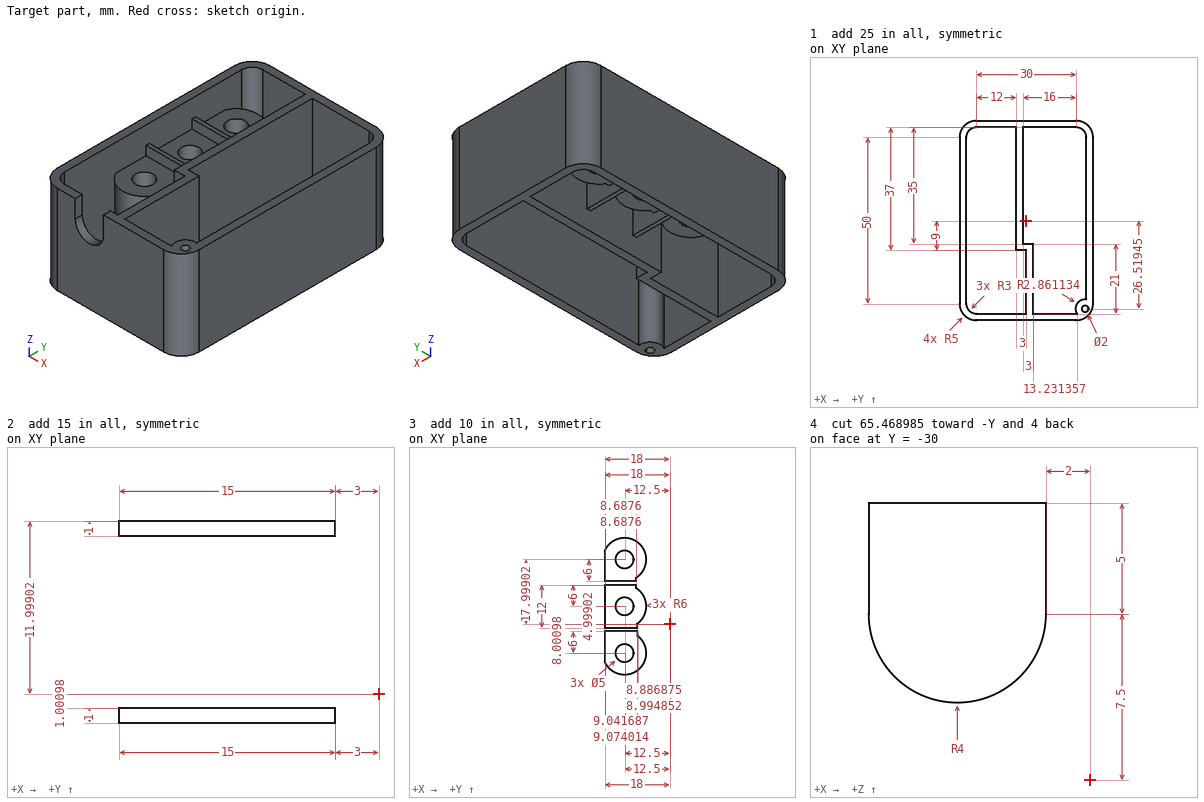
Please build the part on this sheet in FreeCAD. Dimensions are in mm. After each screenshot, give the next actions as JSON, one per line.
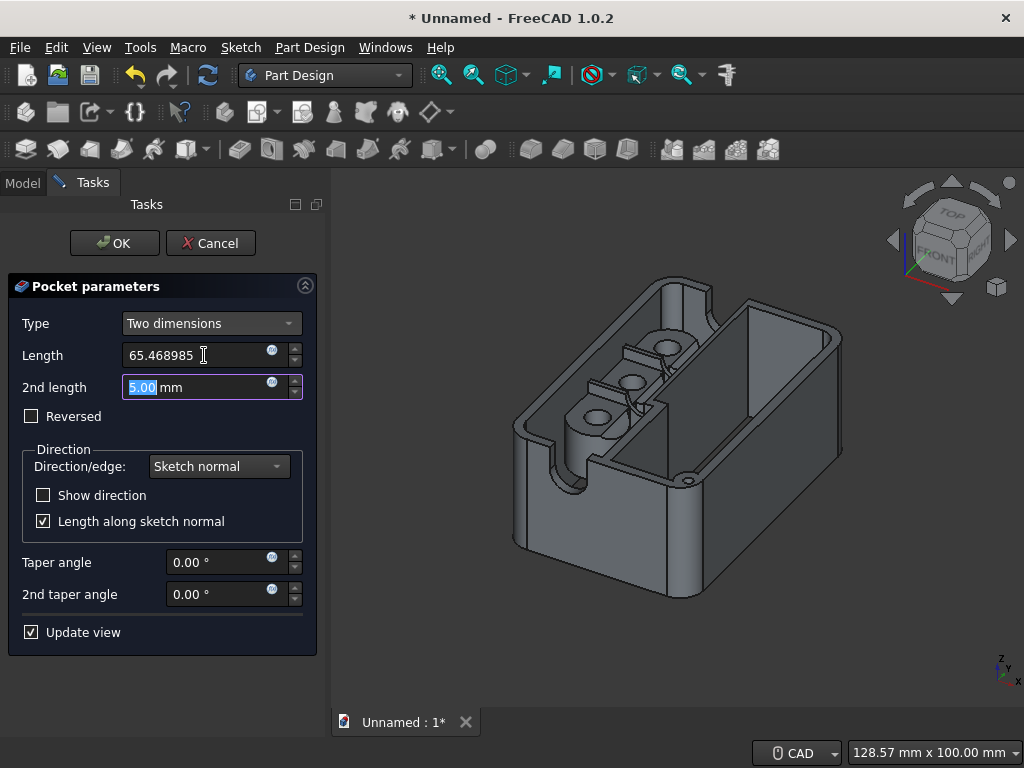
{"action": "type", "text": "4"}
{"action": "key", "text": "Tab"}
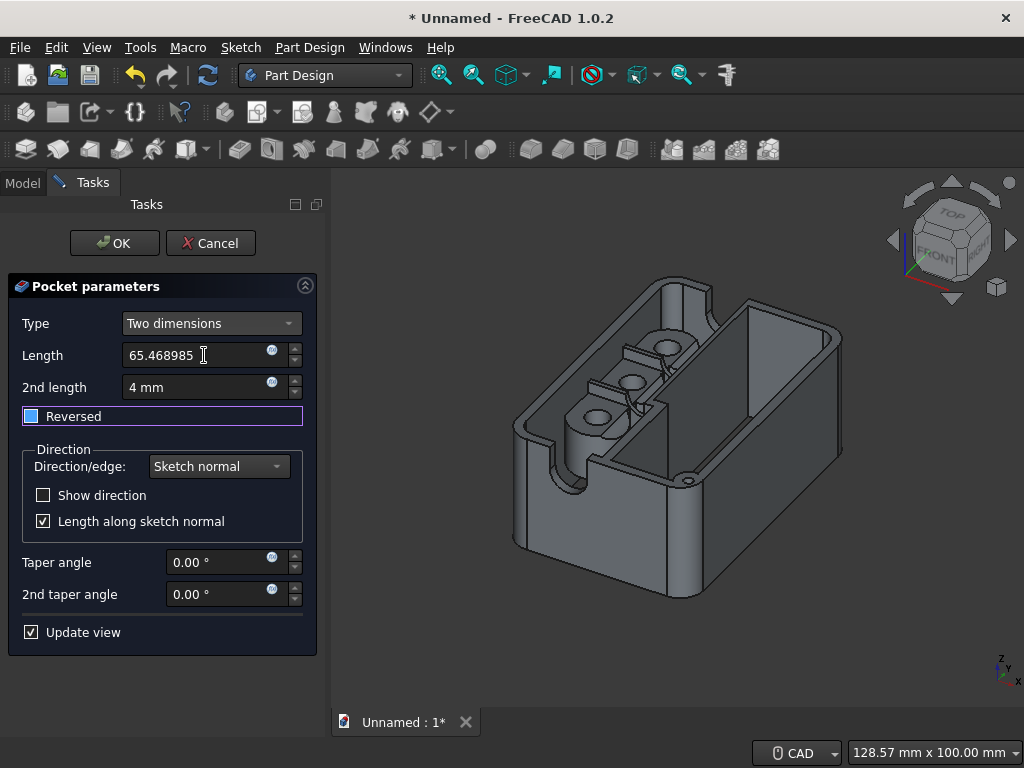
{"action": "left_click", "coordinate": [30, 416]}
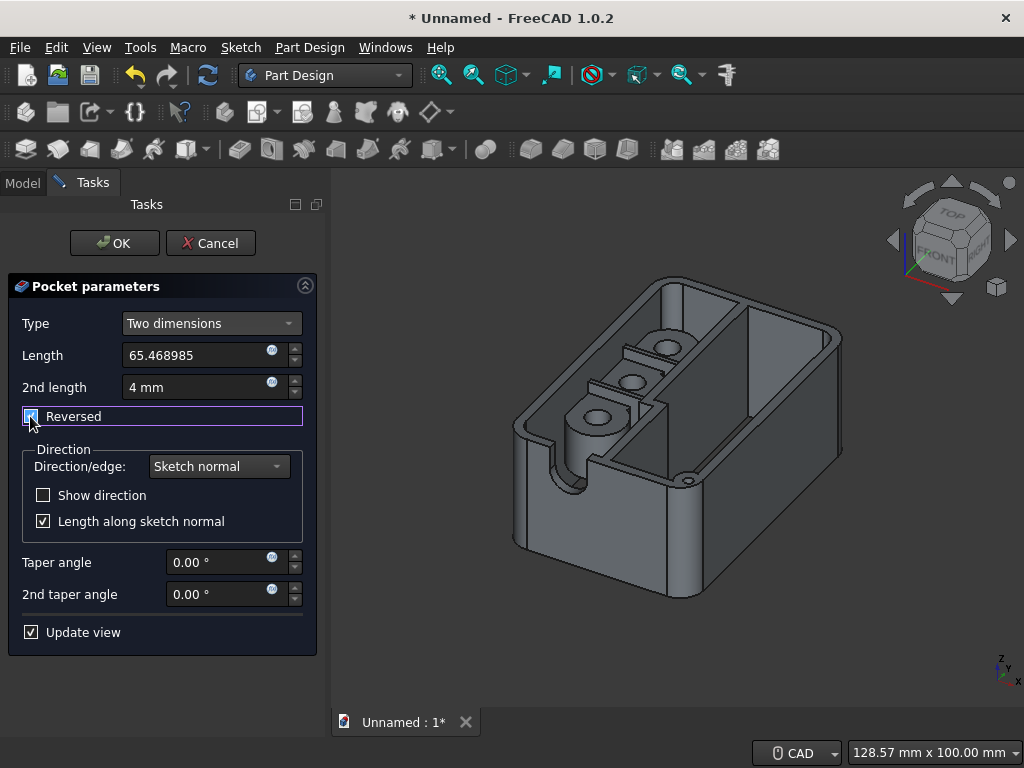
{"action": "left_click", "coordinate": [115, 243]}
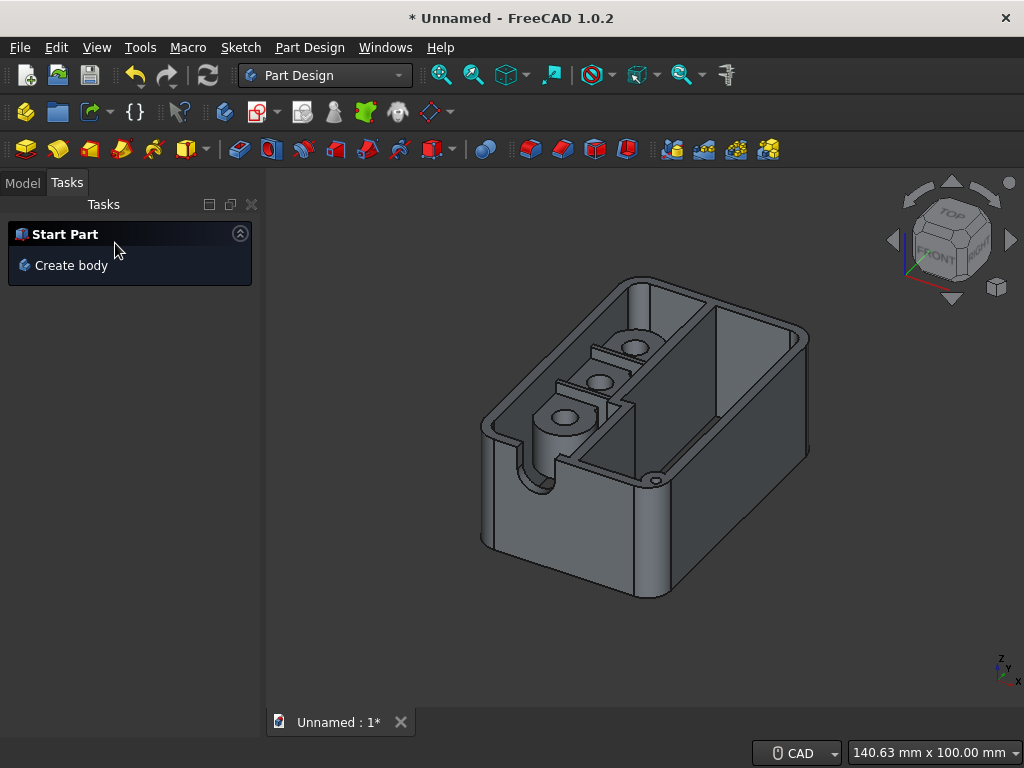
{"action": "key", "text": "0"}